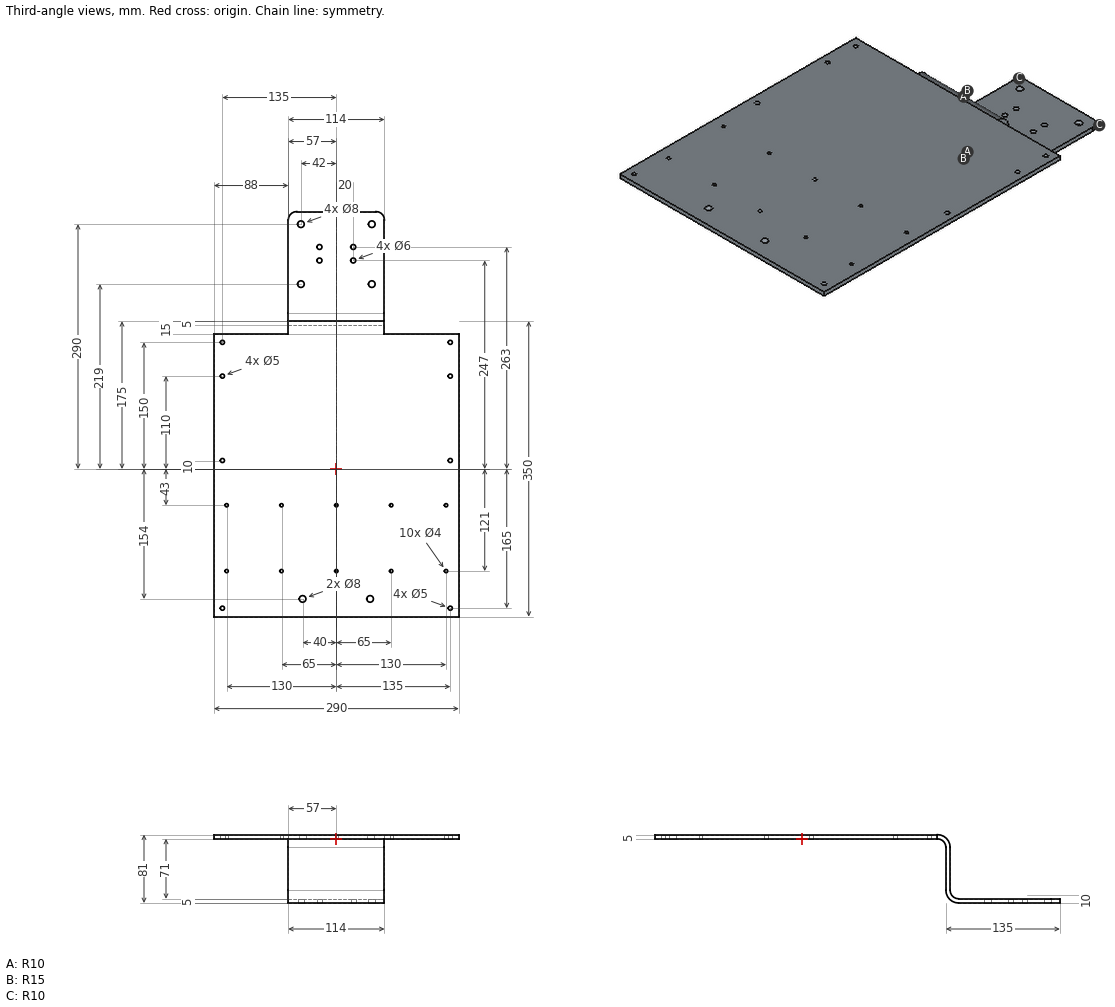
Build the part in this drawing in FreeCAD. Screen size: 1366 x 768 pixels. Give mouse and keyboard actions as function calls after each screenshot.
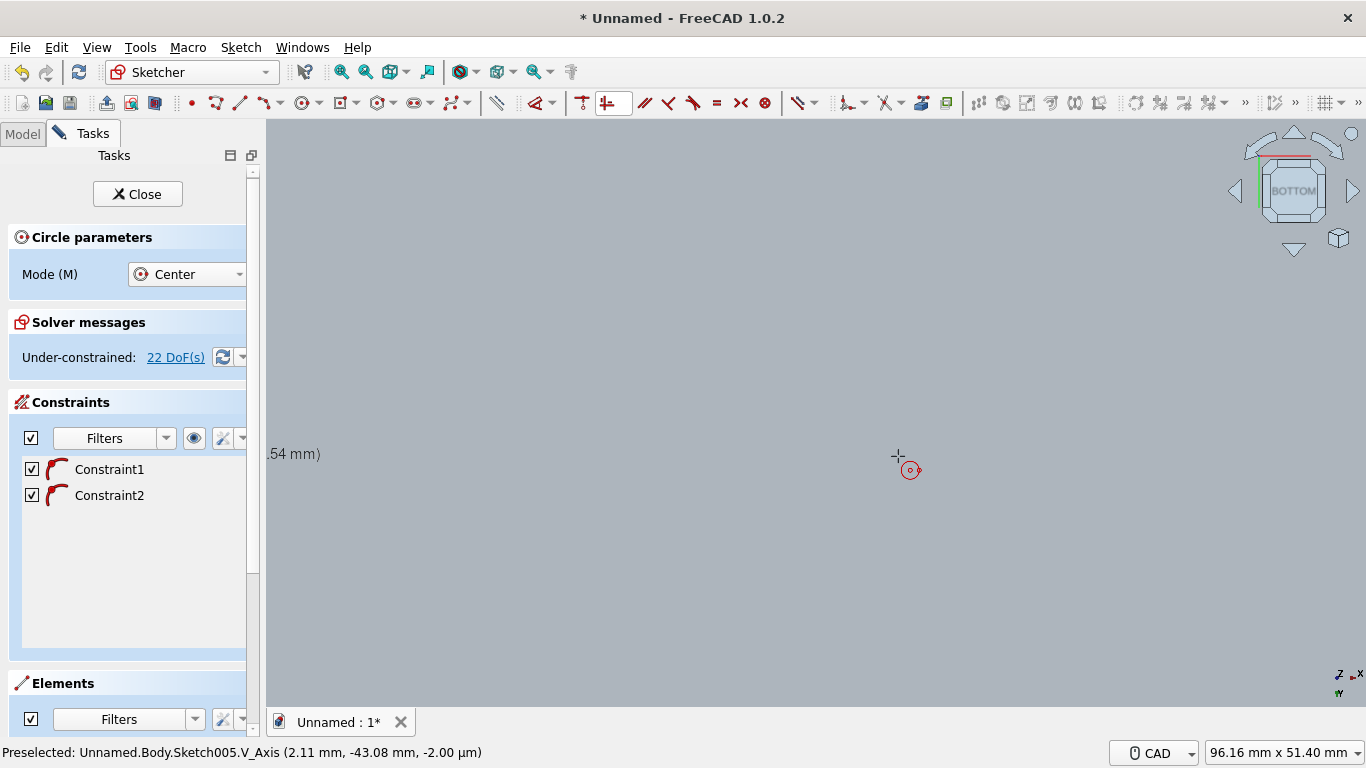
scroll(899, 456, down, 8)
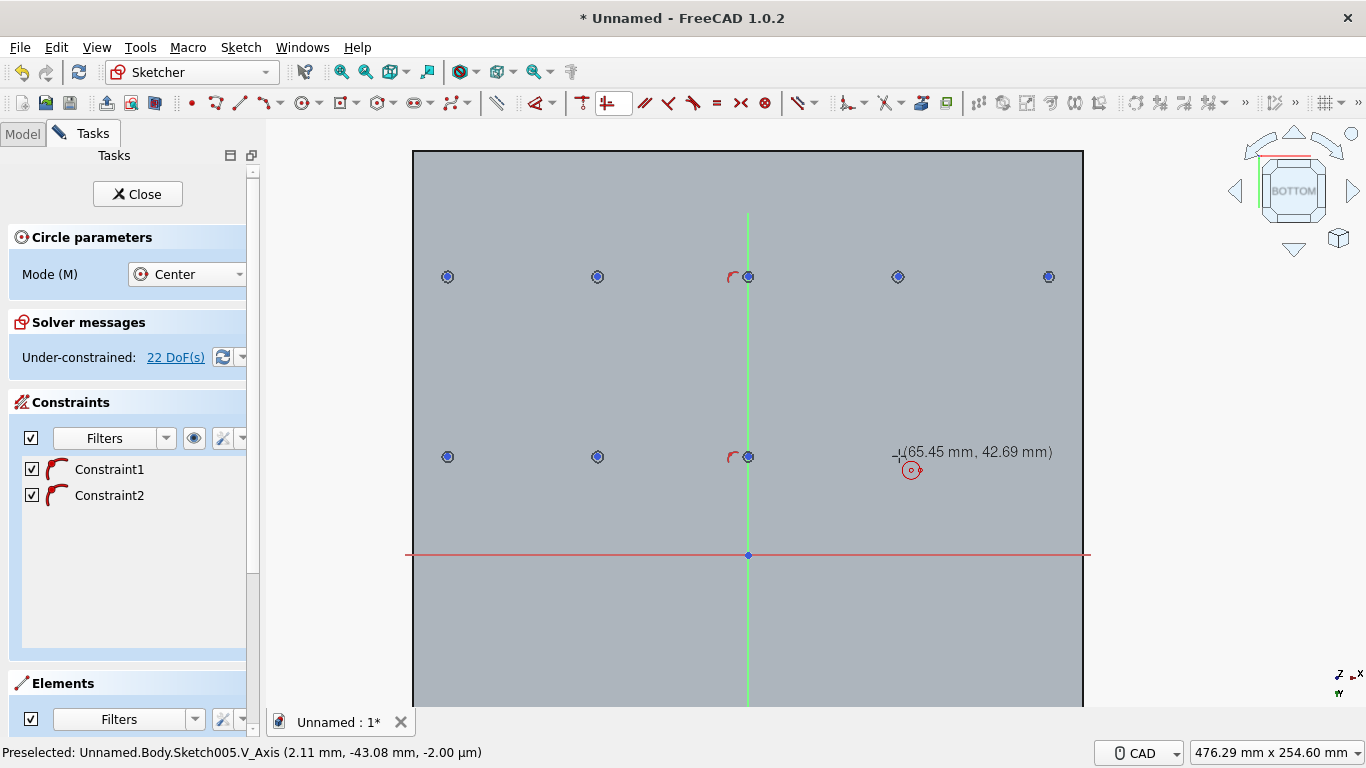
click(898, 456)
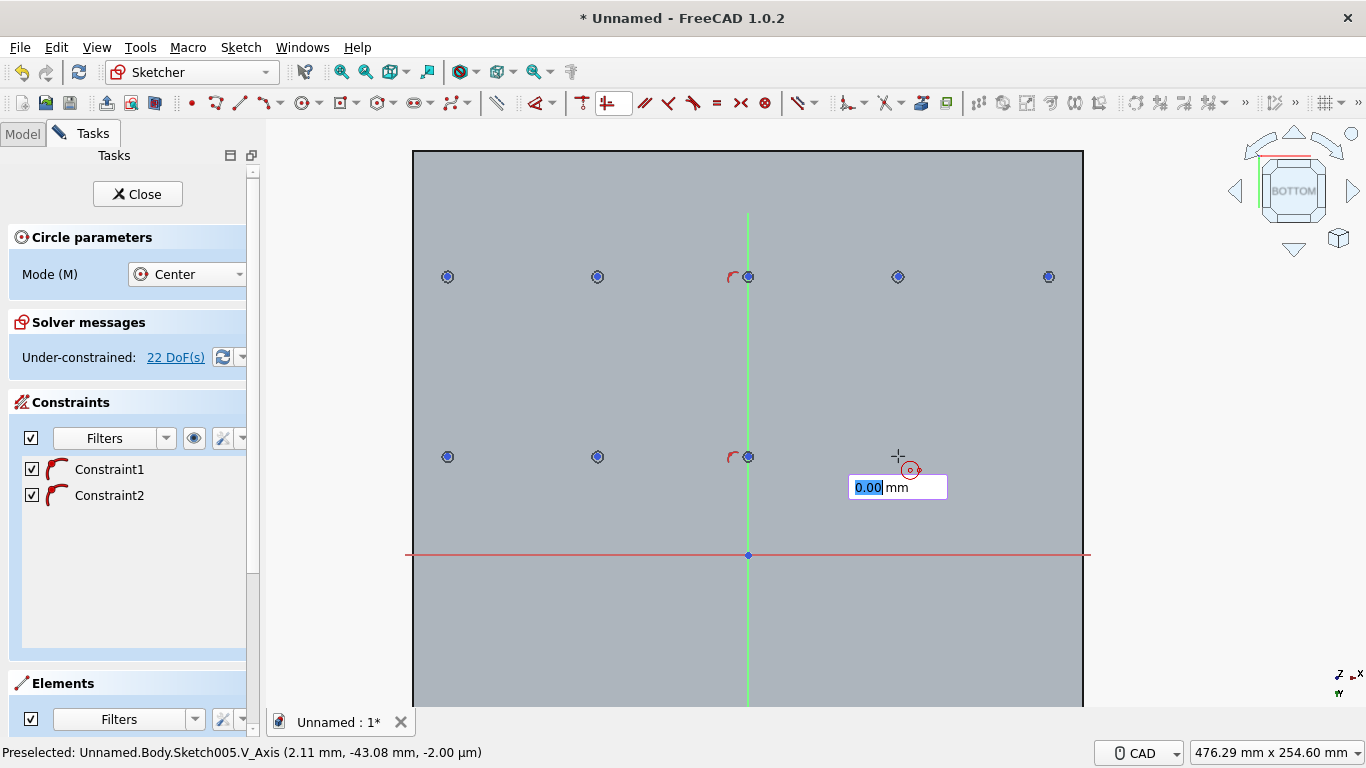
scroll(902, 453, up, 7)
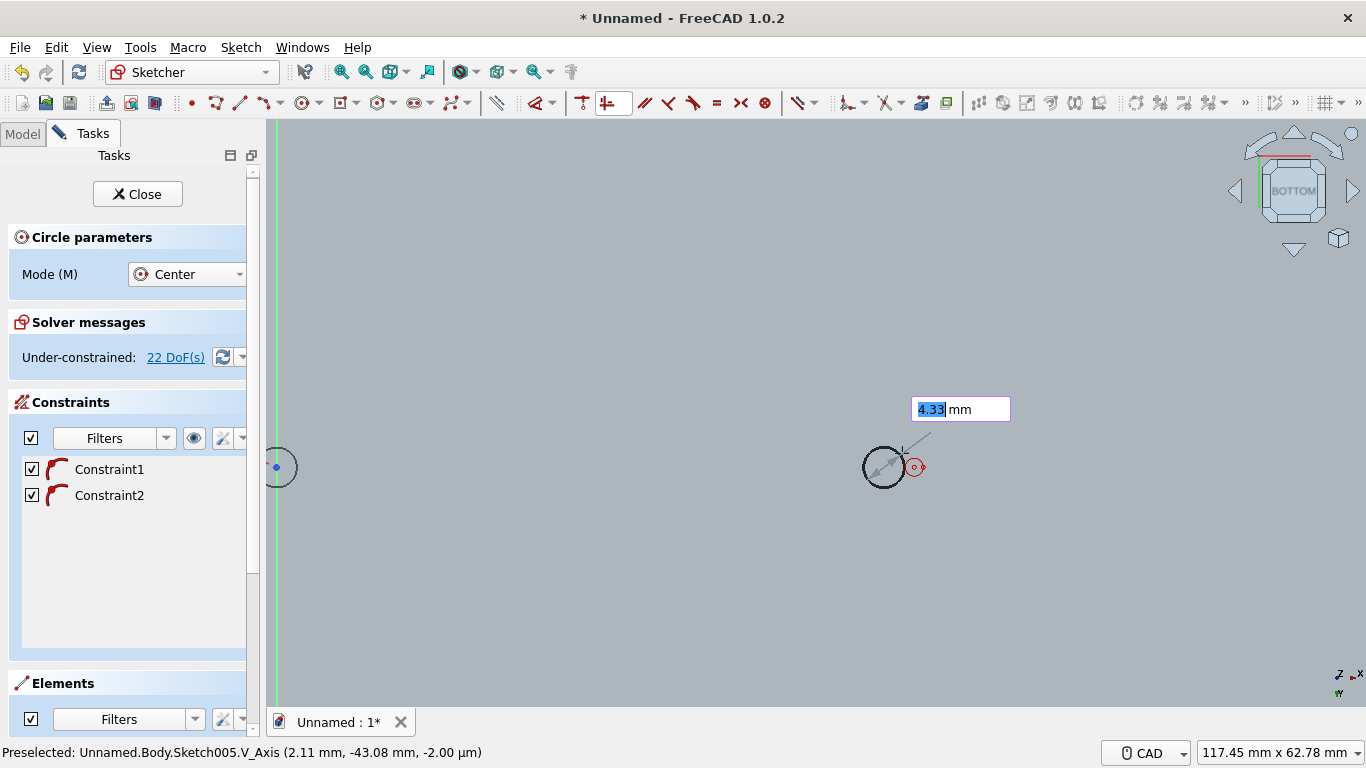
click(899, 450)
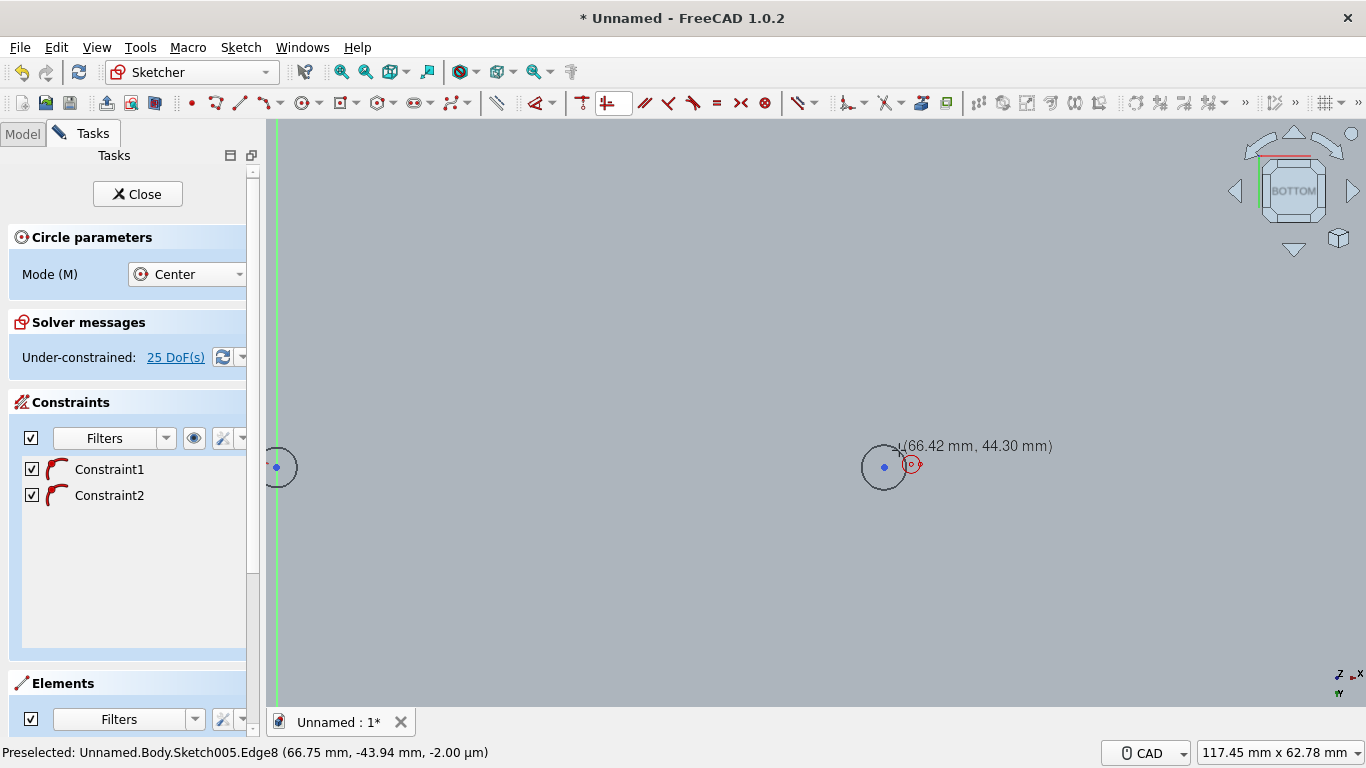
scroll(902, 453, down, 7)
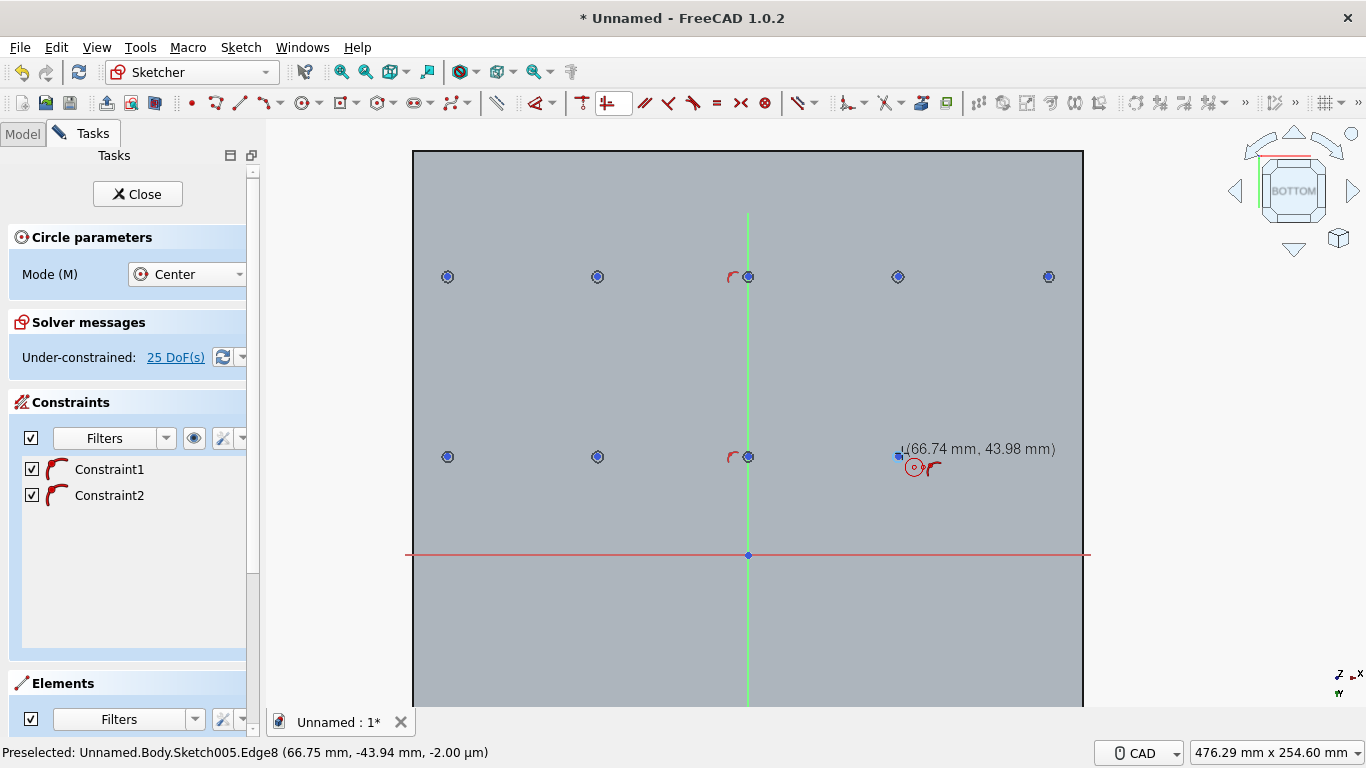
scroll(1049, 456, up, 8)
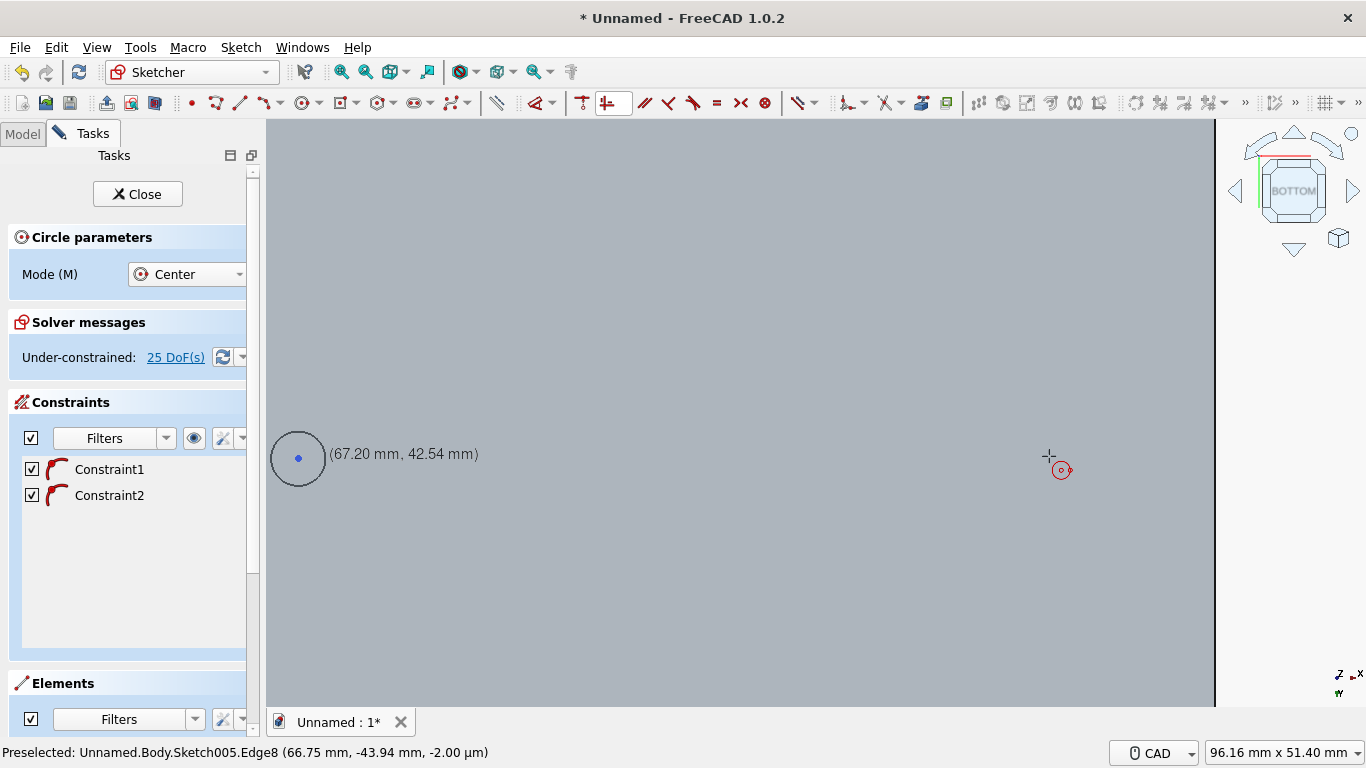
scroll(1049, 456, down, 8)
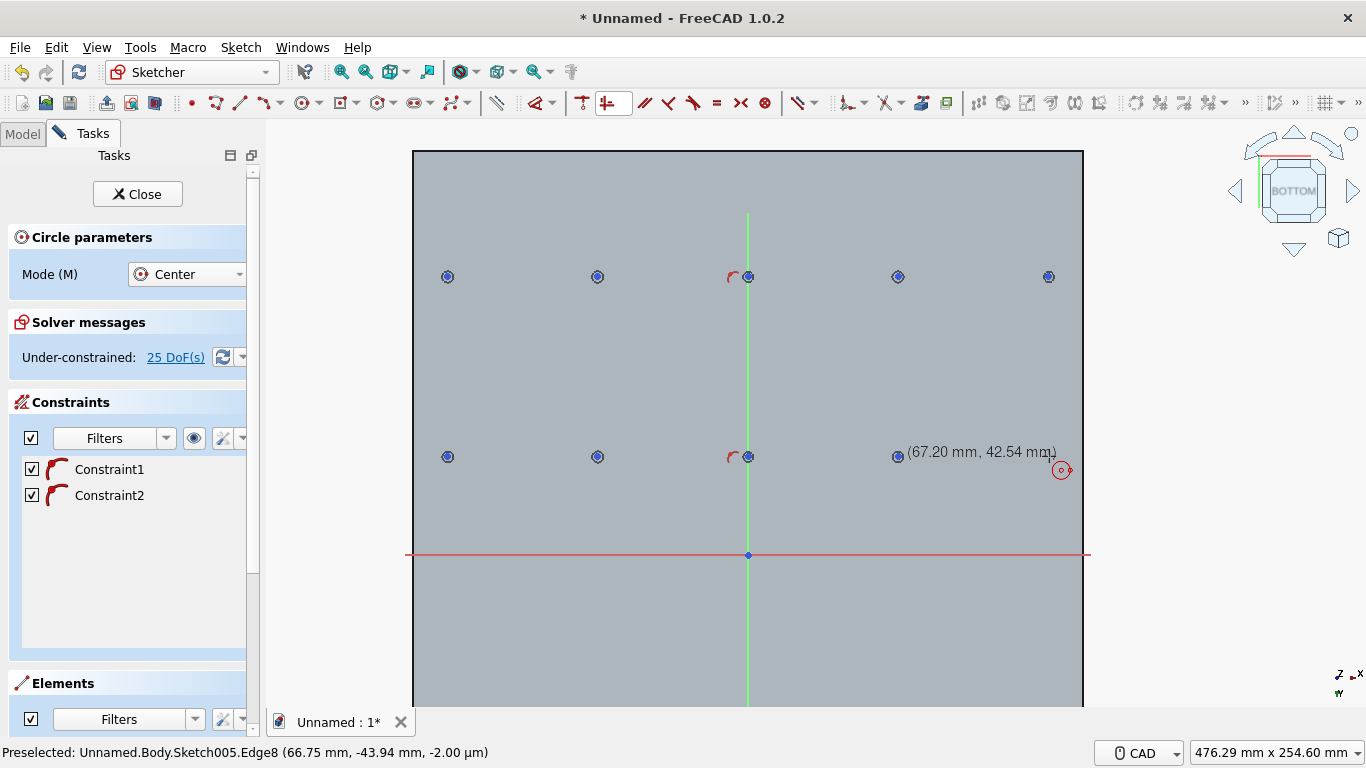
click(1049, 456)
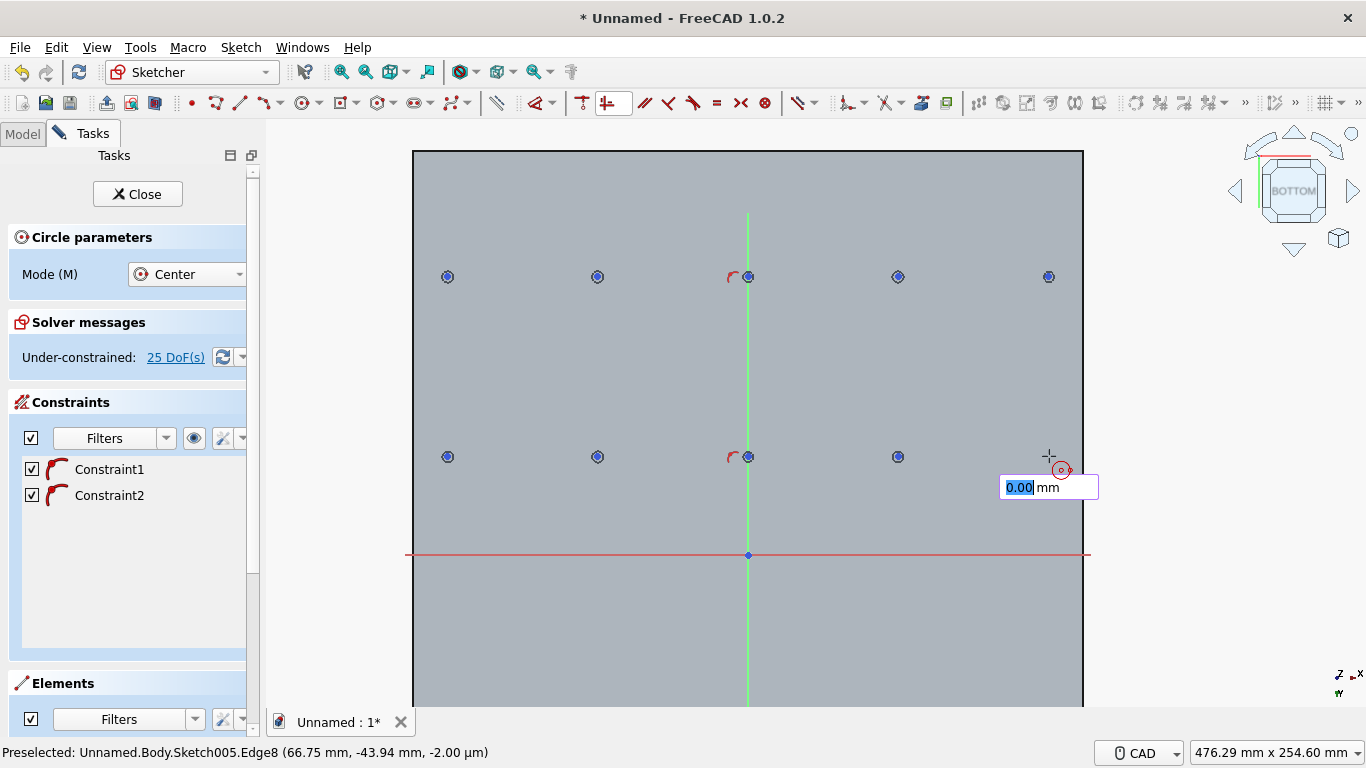
scroll(1052, 453, up, 7)